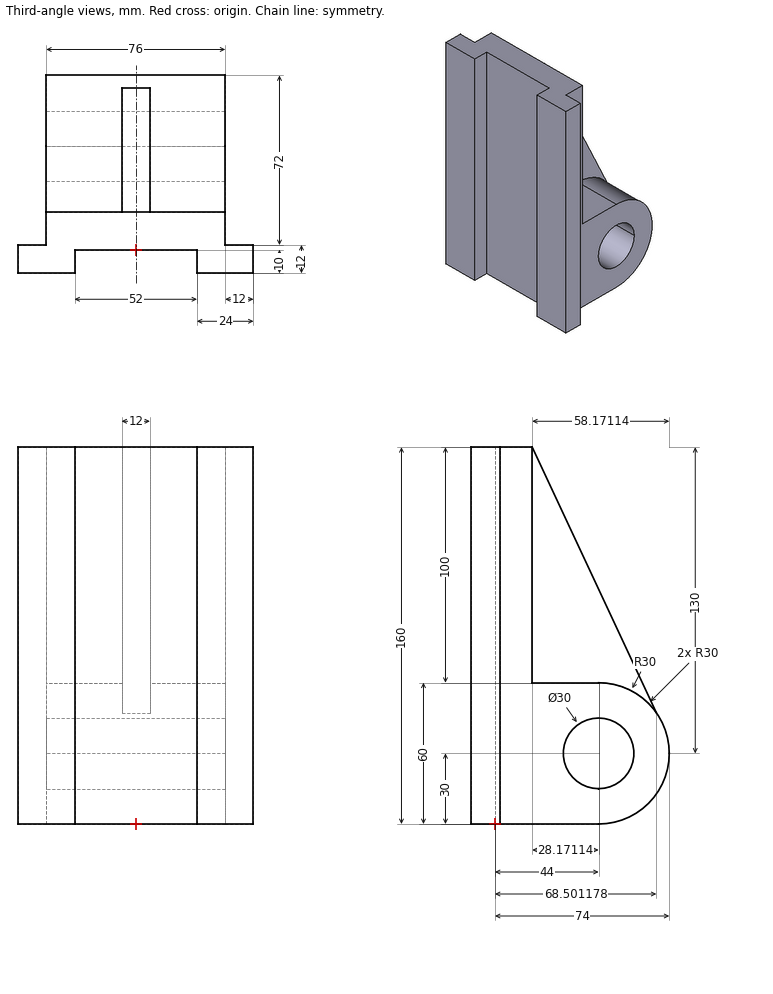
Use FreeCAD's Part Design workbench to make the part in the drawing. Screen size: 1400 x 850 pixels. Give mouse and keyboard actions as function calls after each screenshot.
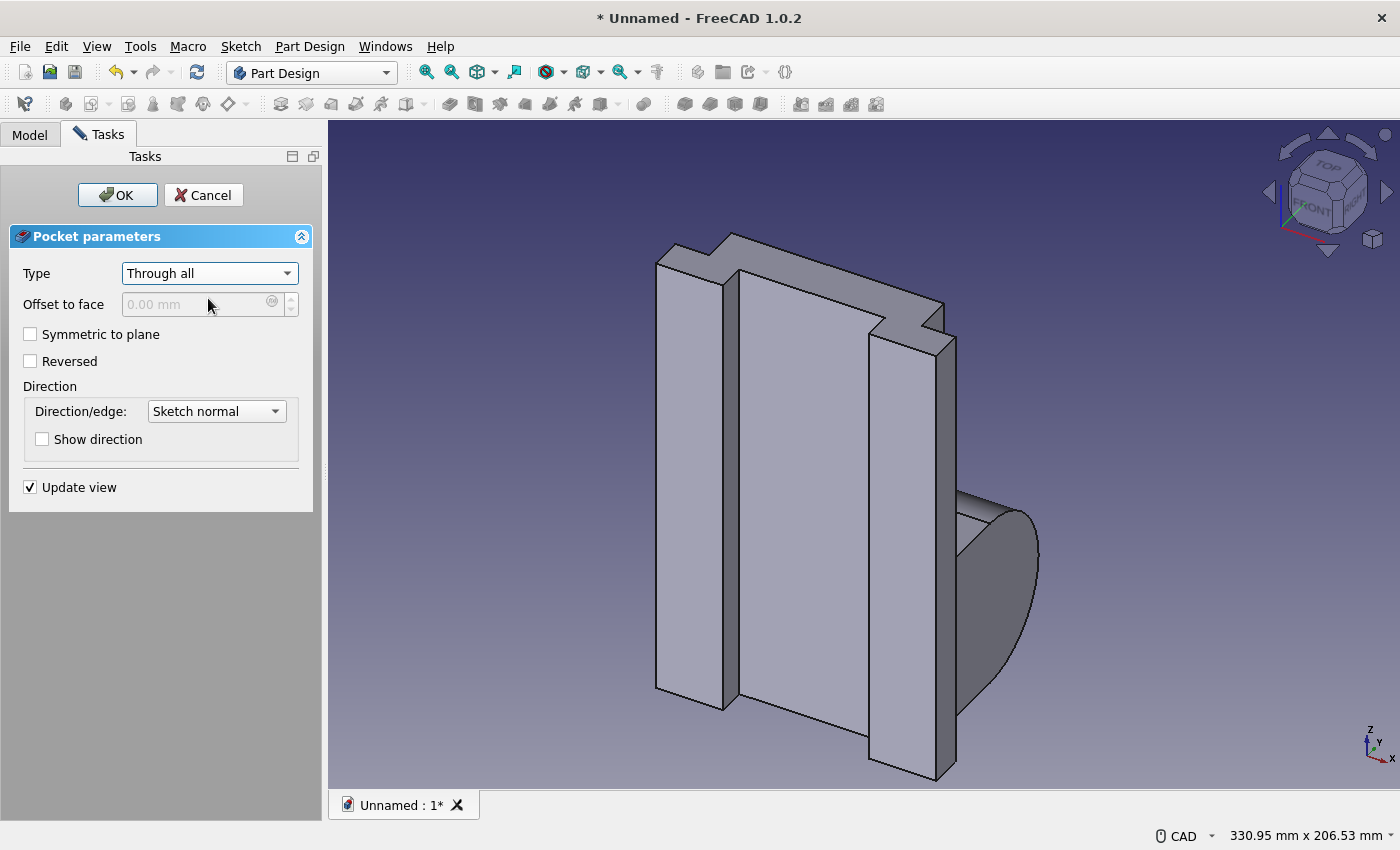
click(118, 195)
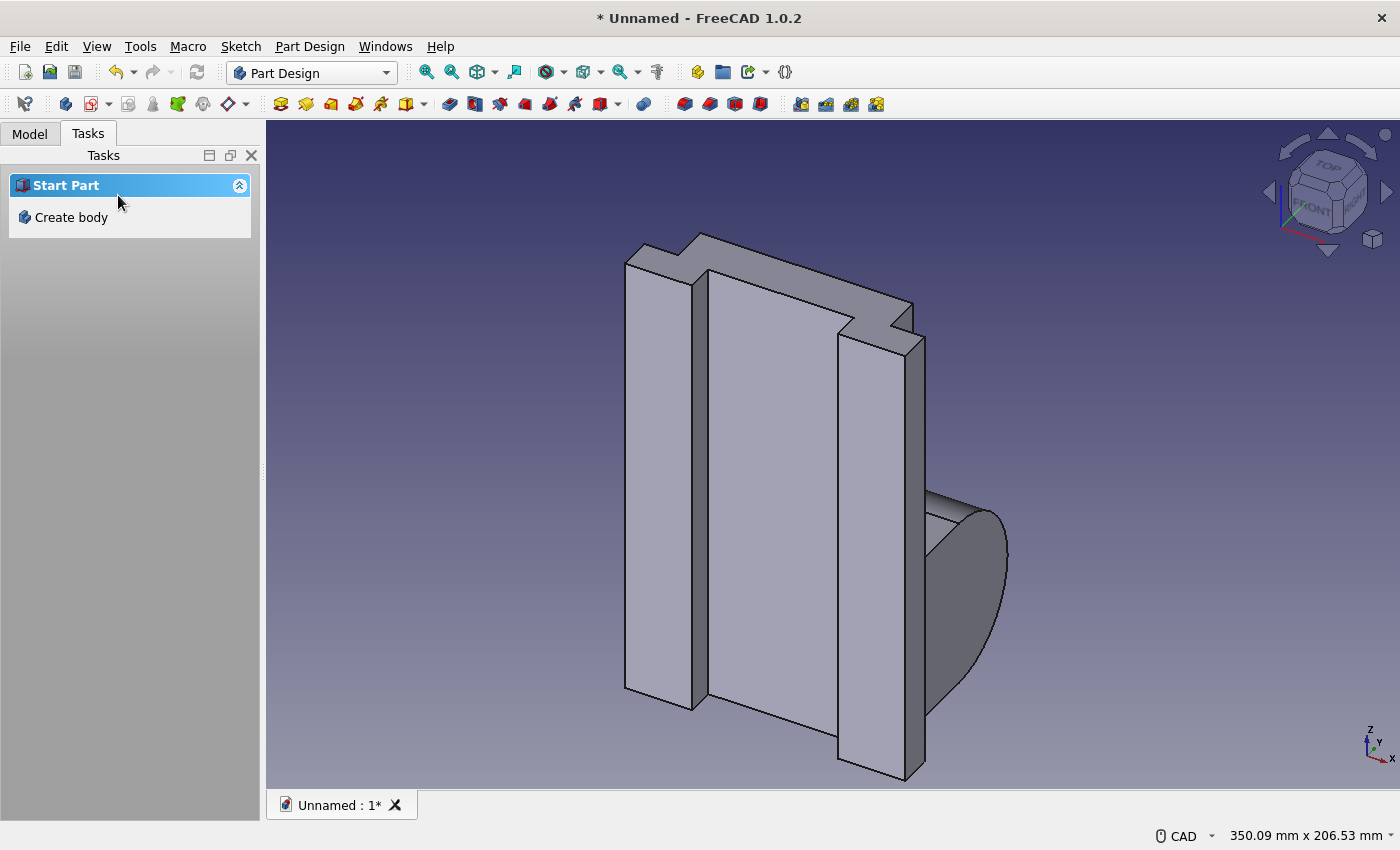
click(90, 104)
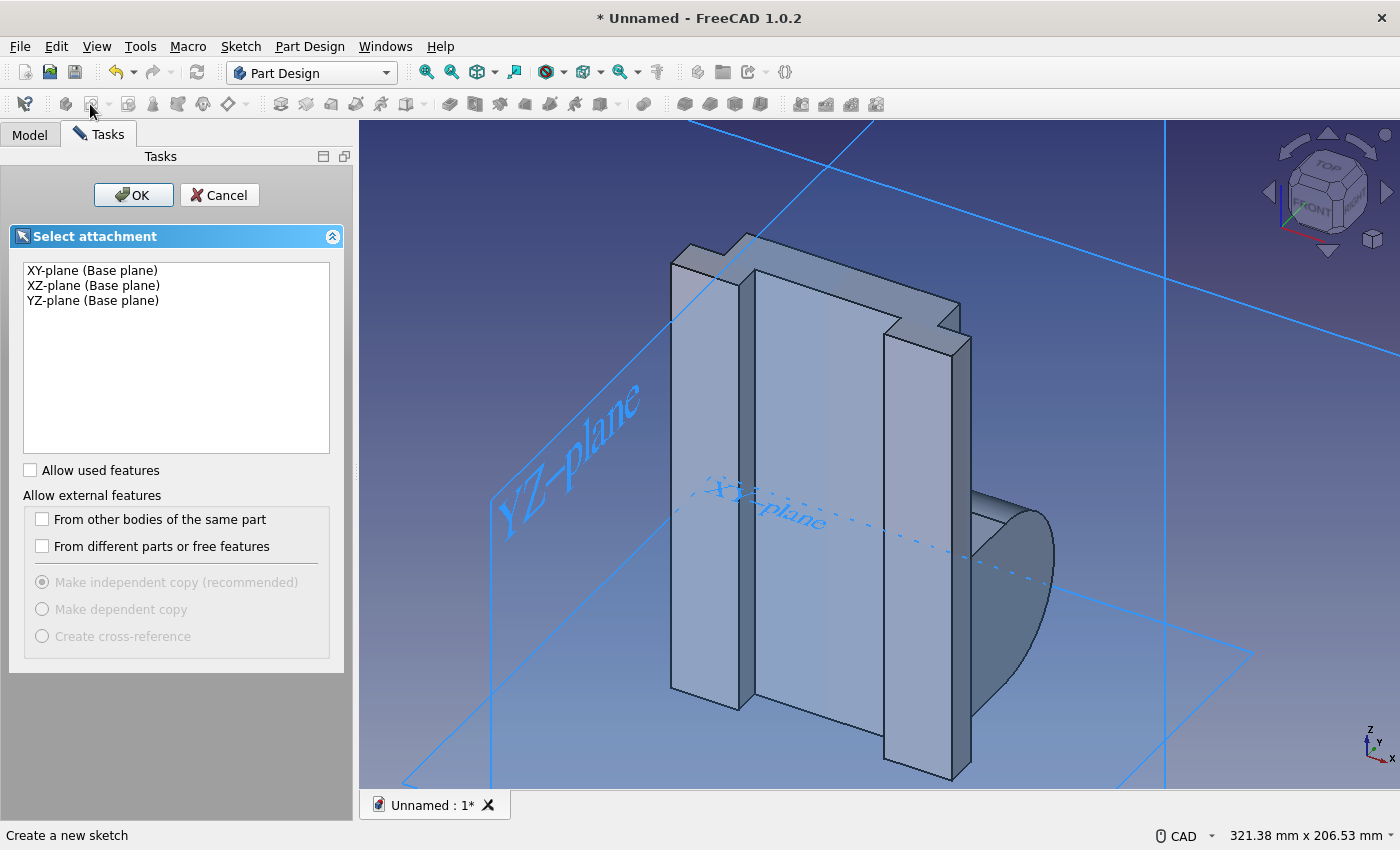
click(84, 300)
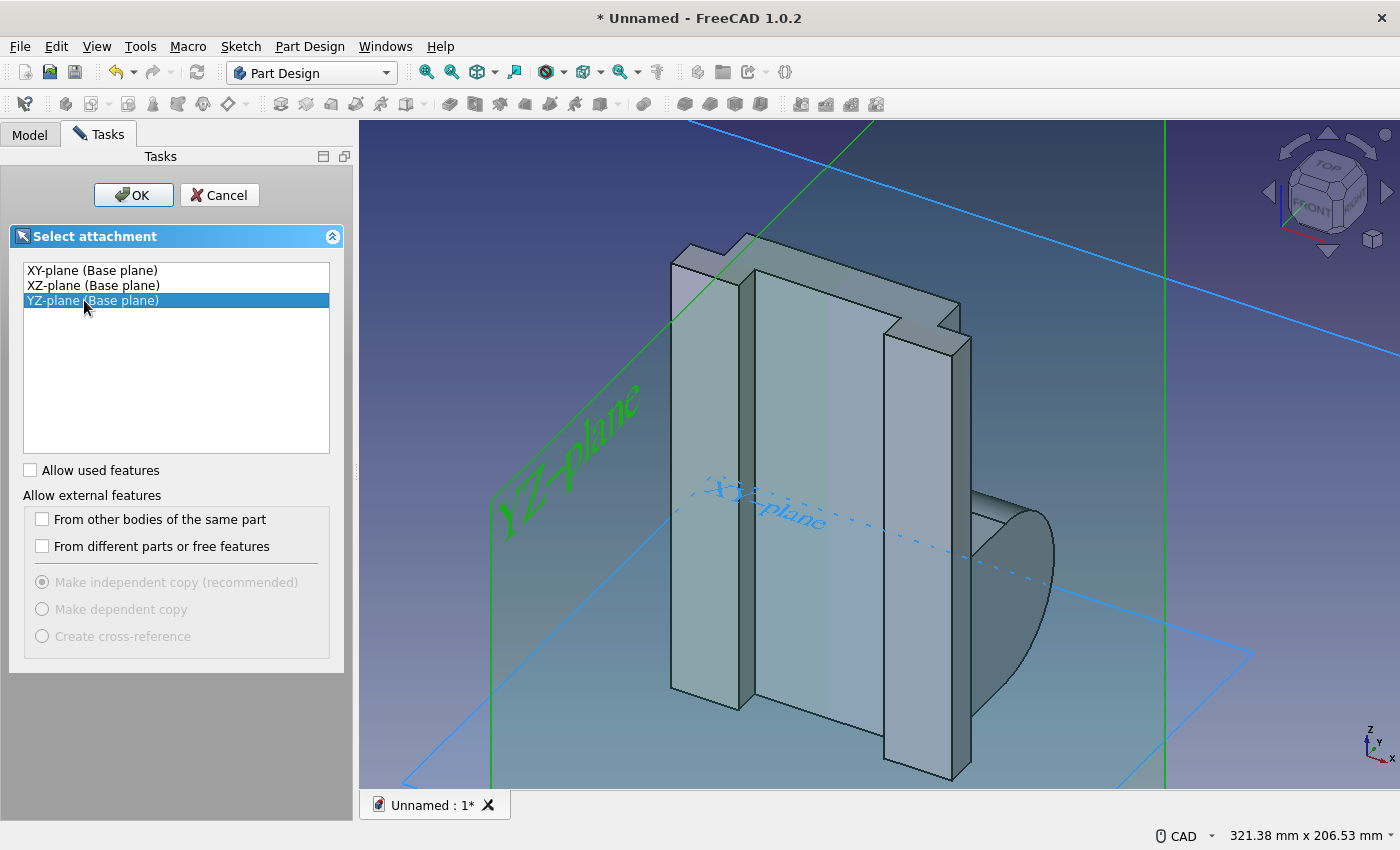
click(134, 195)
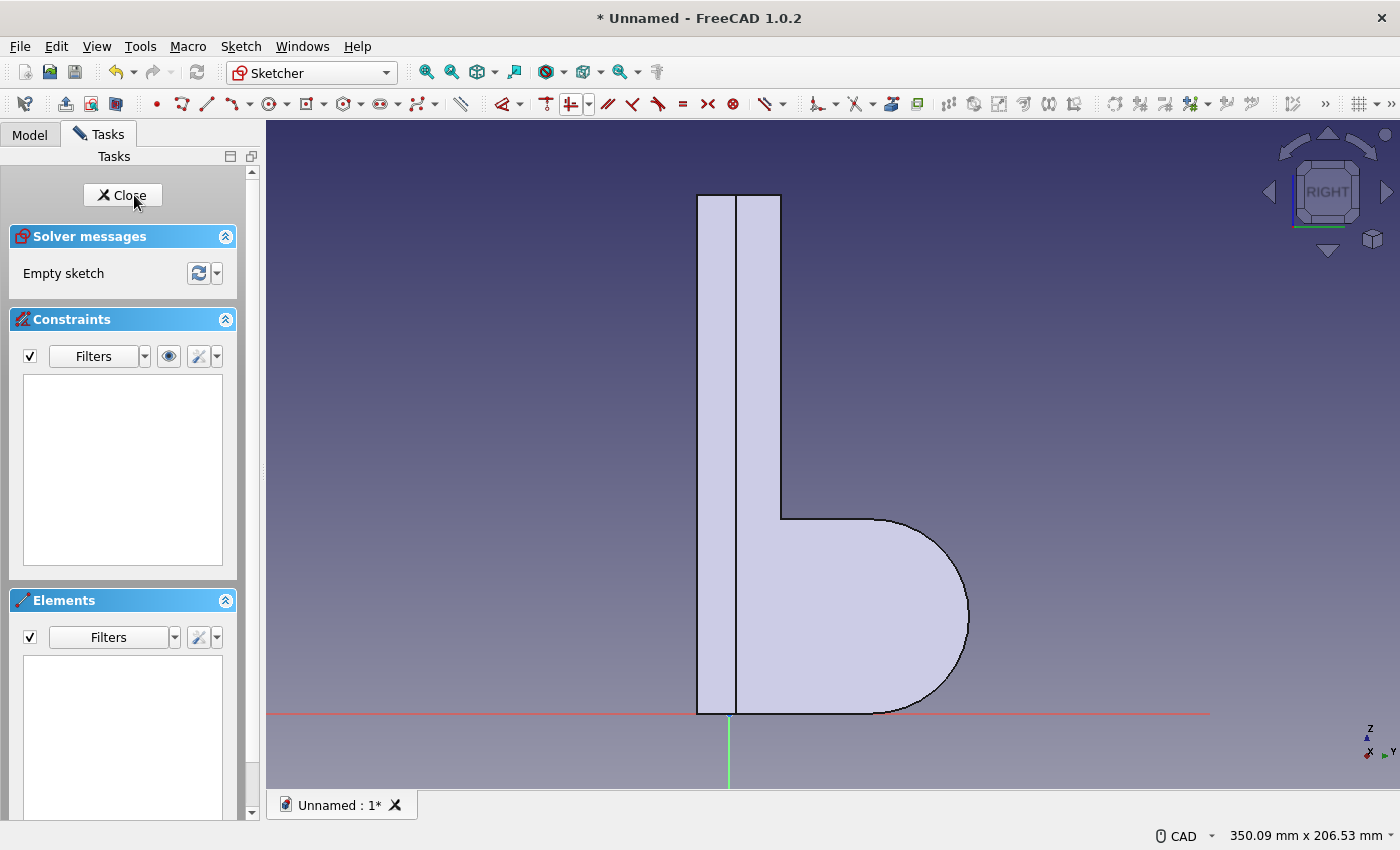
key(q)
key(s)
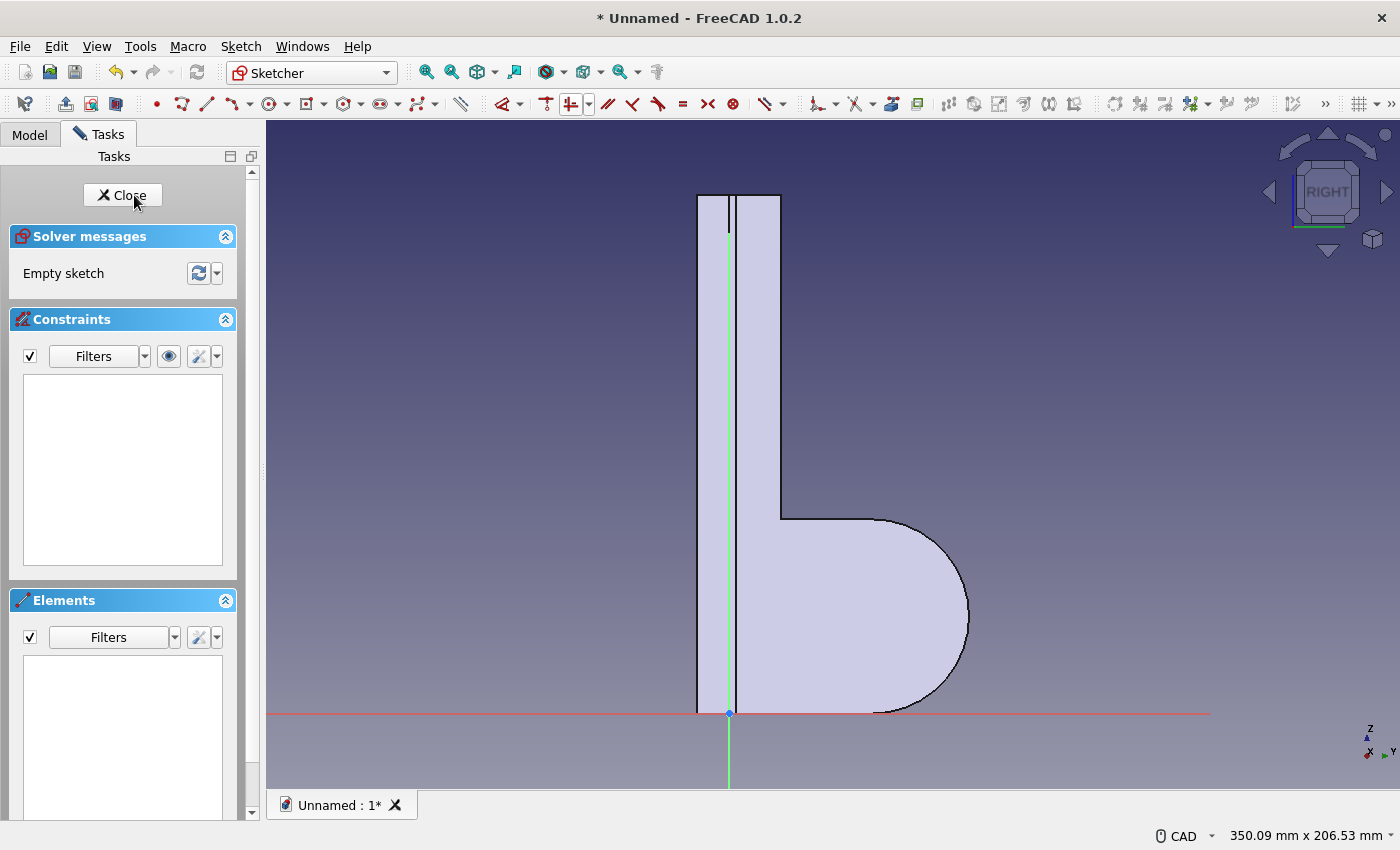
key(g)
key(m)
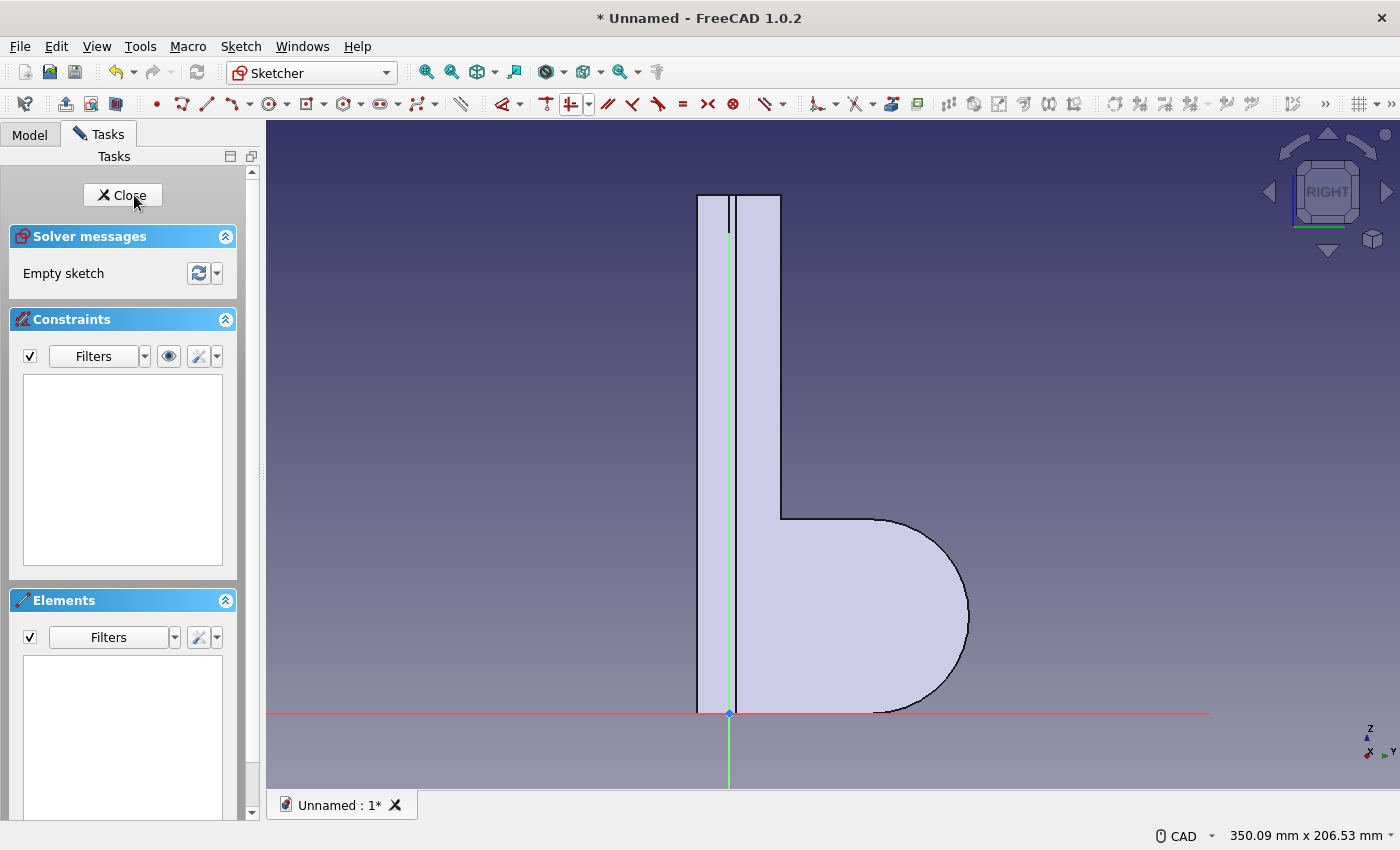
click(951, 560)
click(781, 195)
click(781, 519)
click(872, 519)
right_click(872, 519)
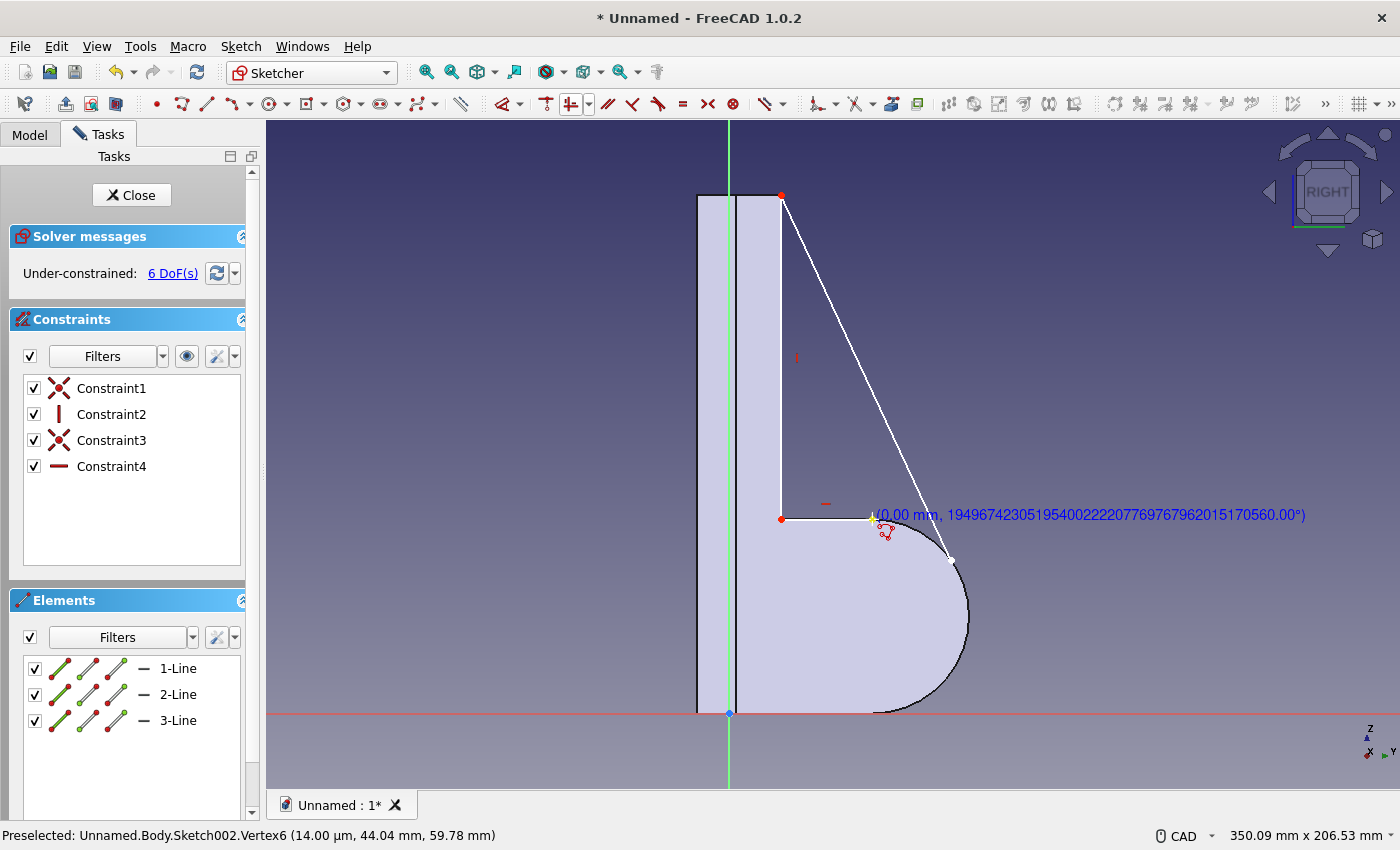
click(232, 104)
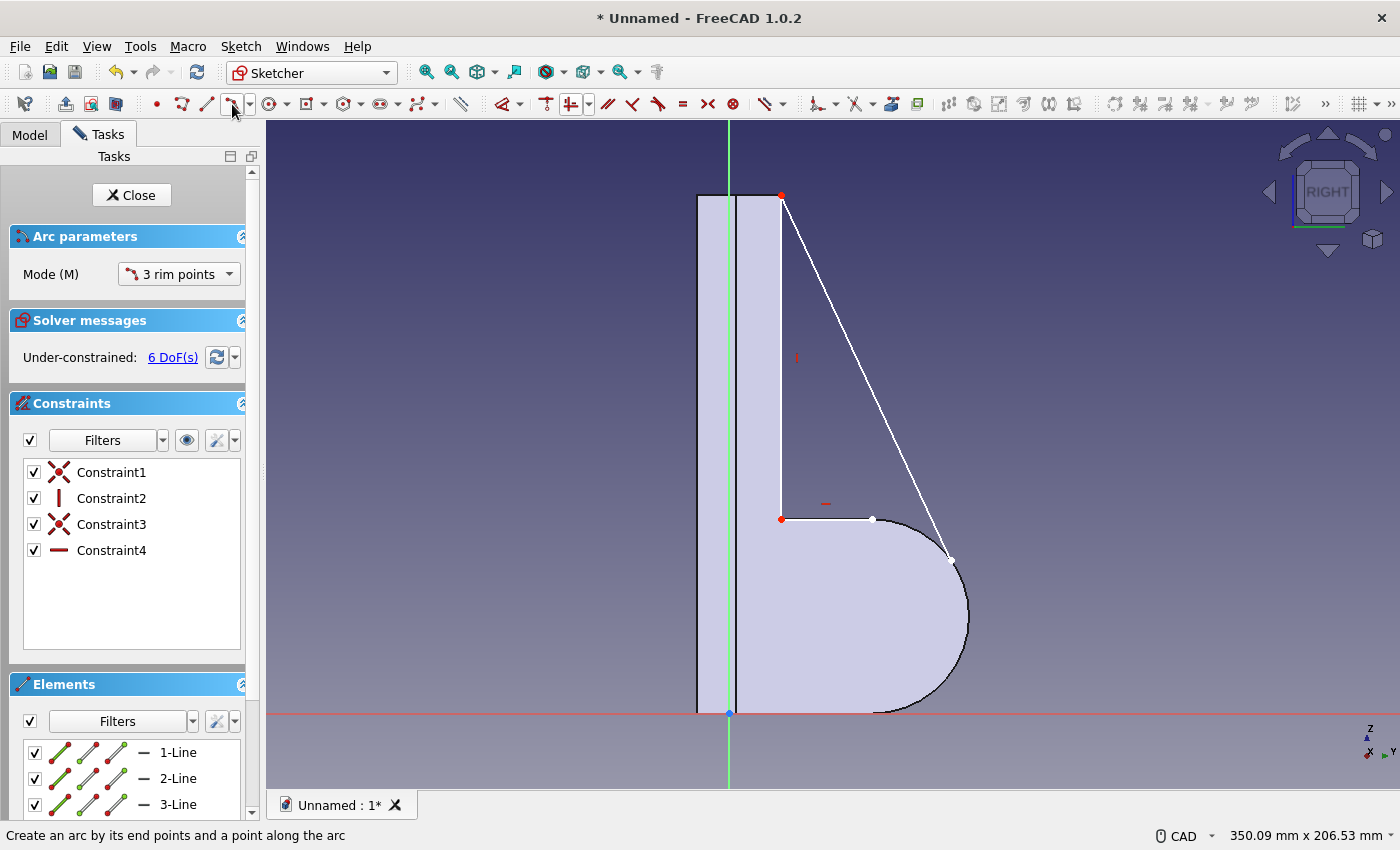
click(872, 520)
click(951, 561)